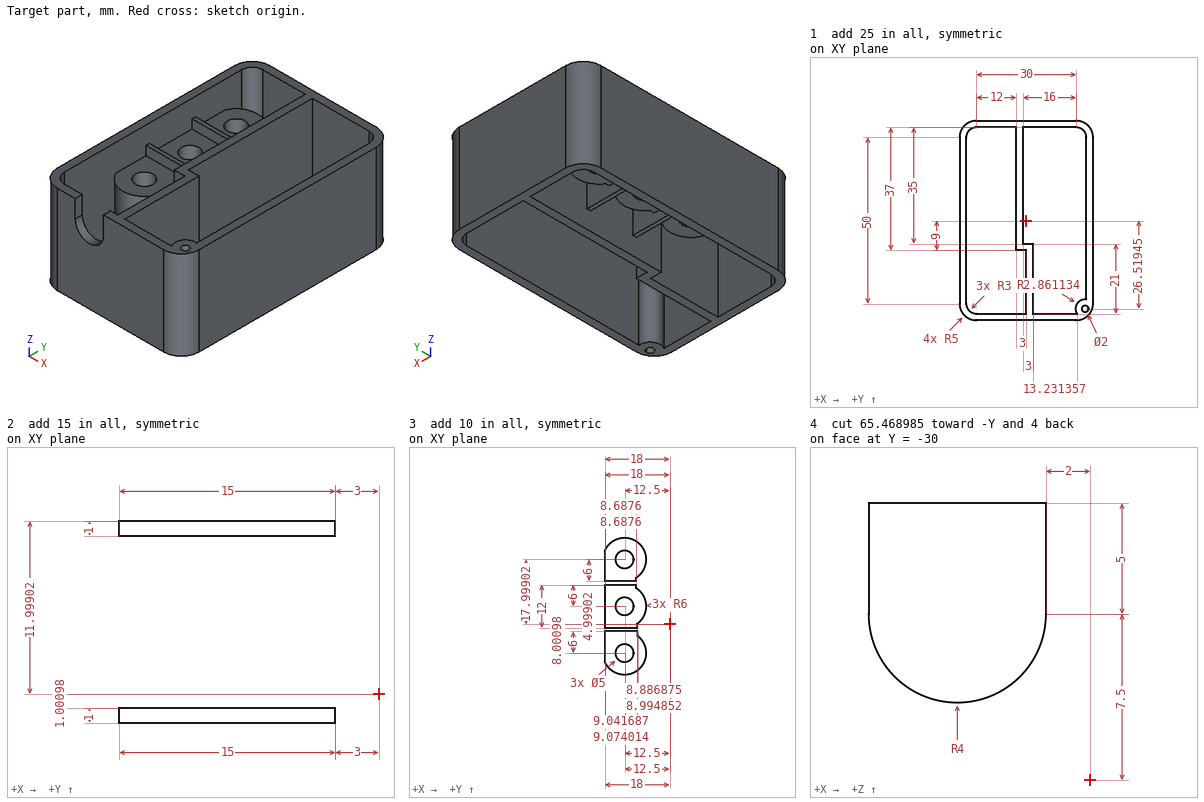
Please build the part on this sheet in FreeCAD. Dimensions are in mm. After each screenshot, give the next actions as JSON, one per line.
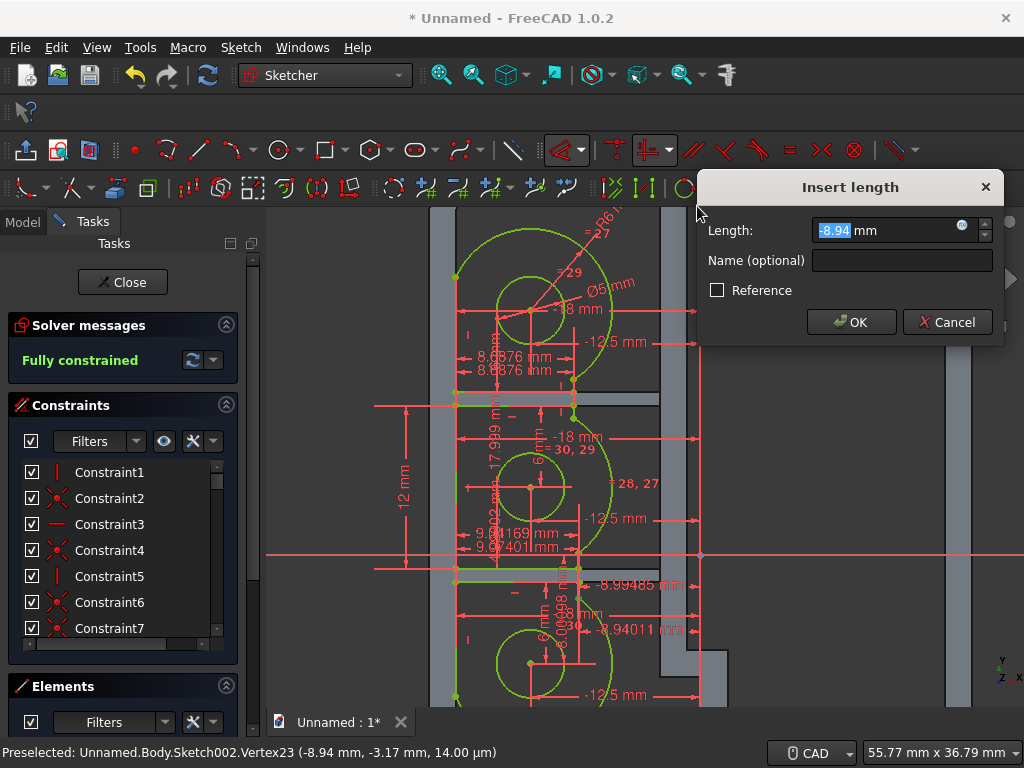
{"action": "type", "text": "-8.886875"}
{"action": "key", "text": "Return"}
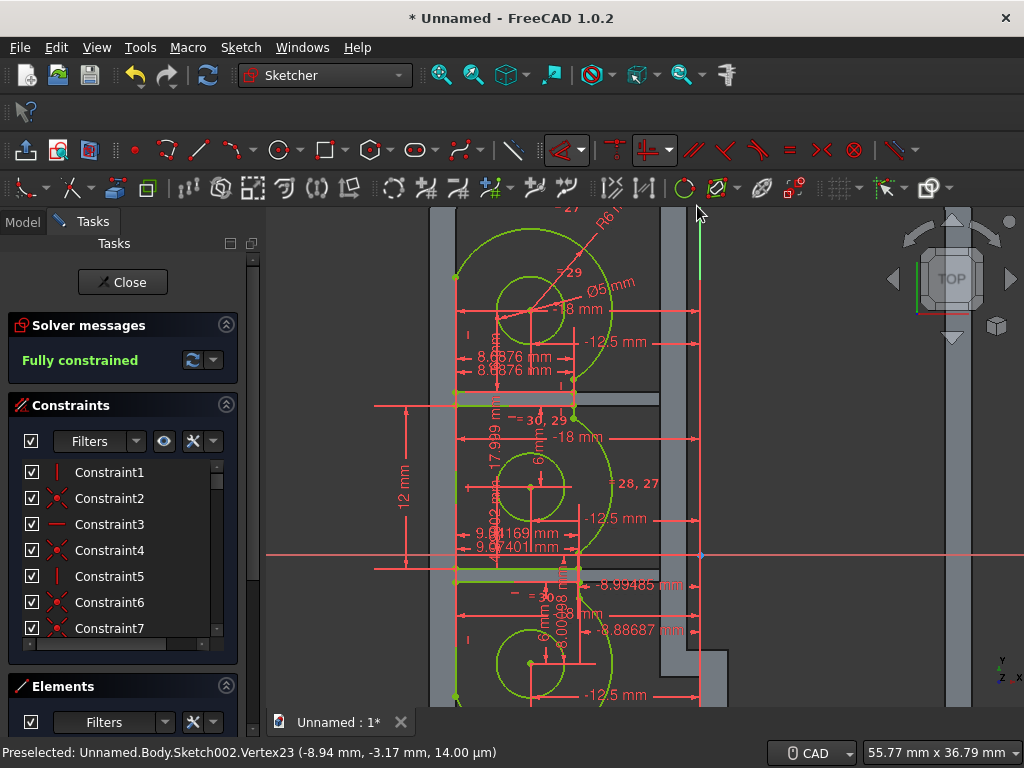
{"action": "left_click", "coordinate": [123, 282]}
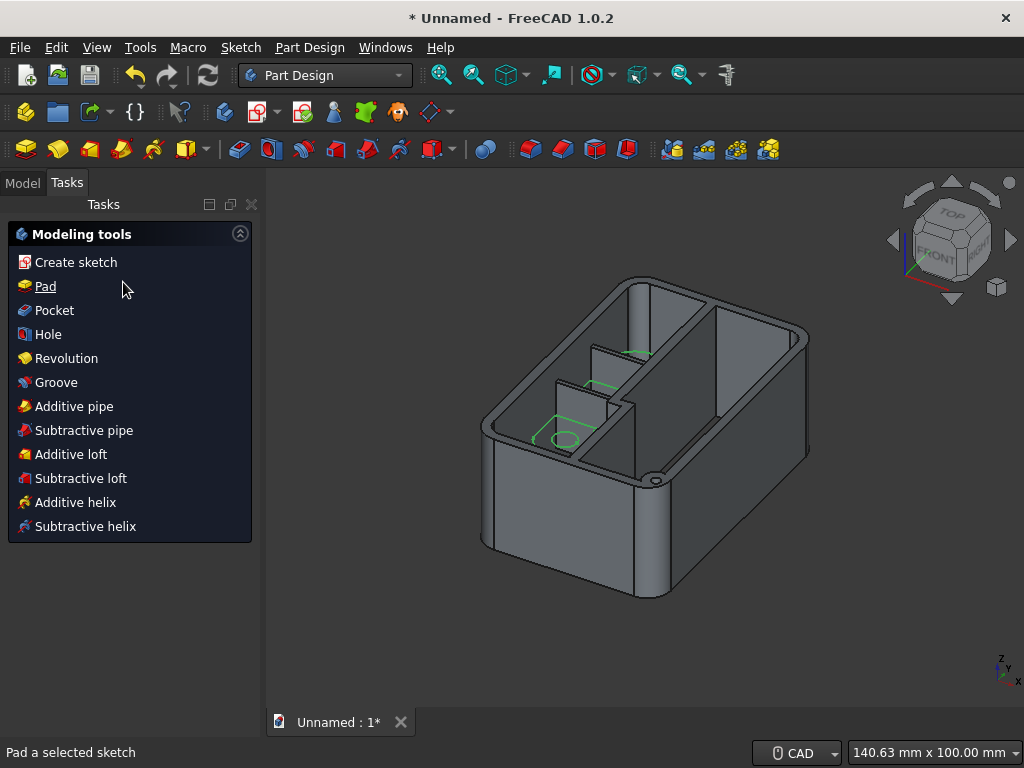
{"action": "left_click", "coordinate": [26, 150]}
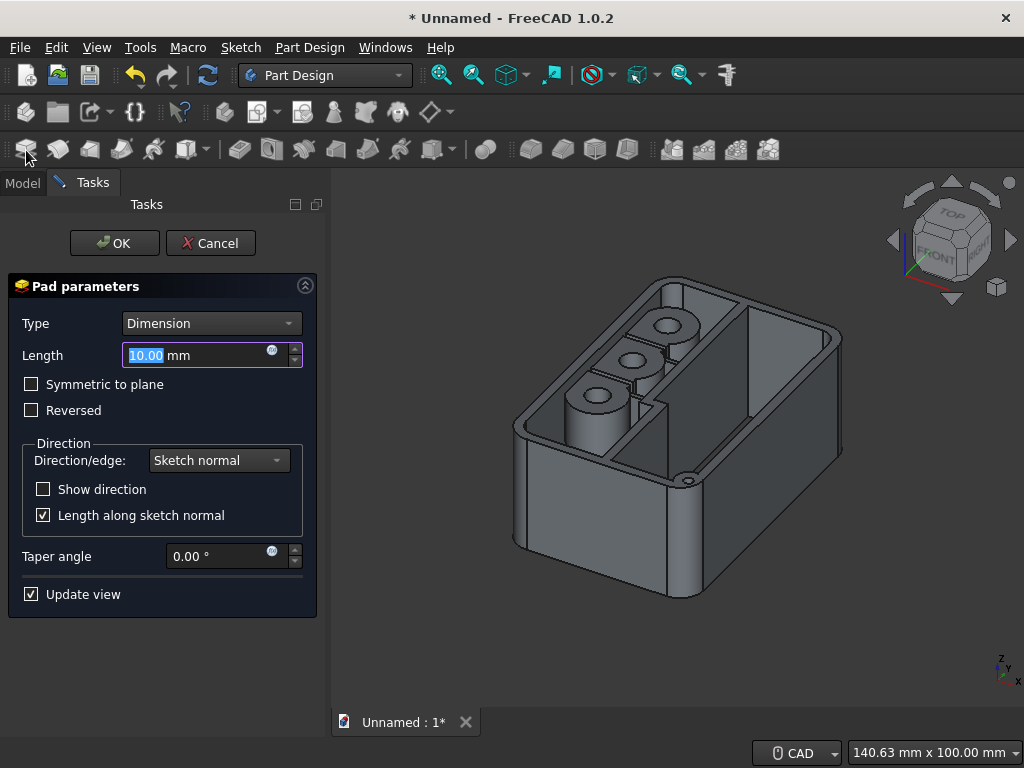
{"action": "type", "text": "10"}
{"action": "key", "text": "Tab"}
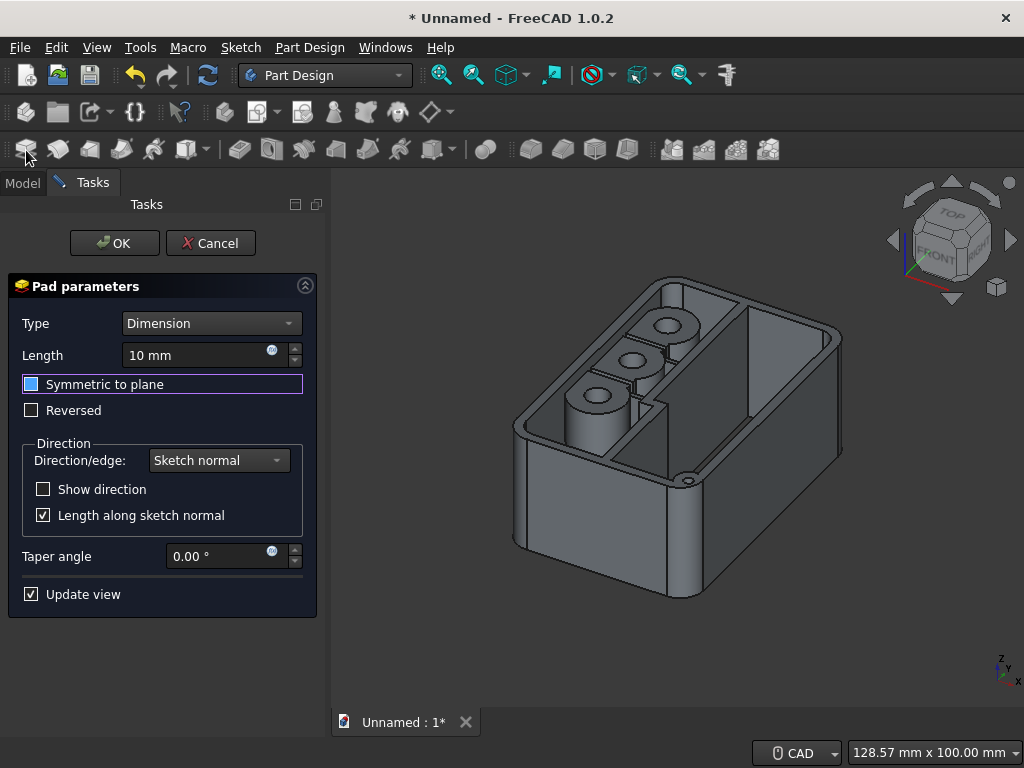
{"action": "left_click", "coordinate": [30, 384]}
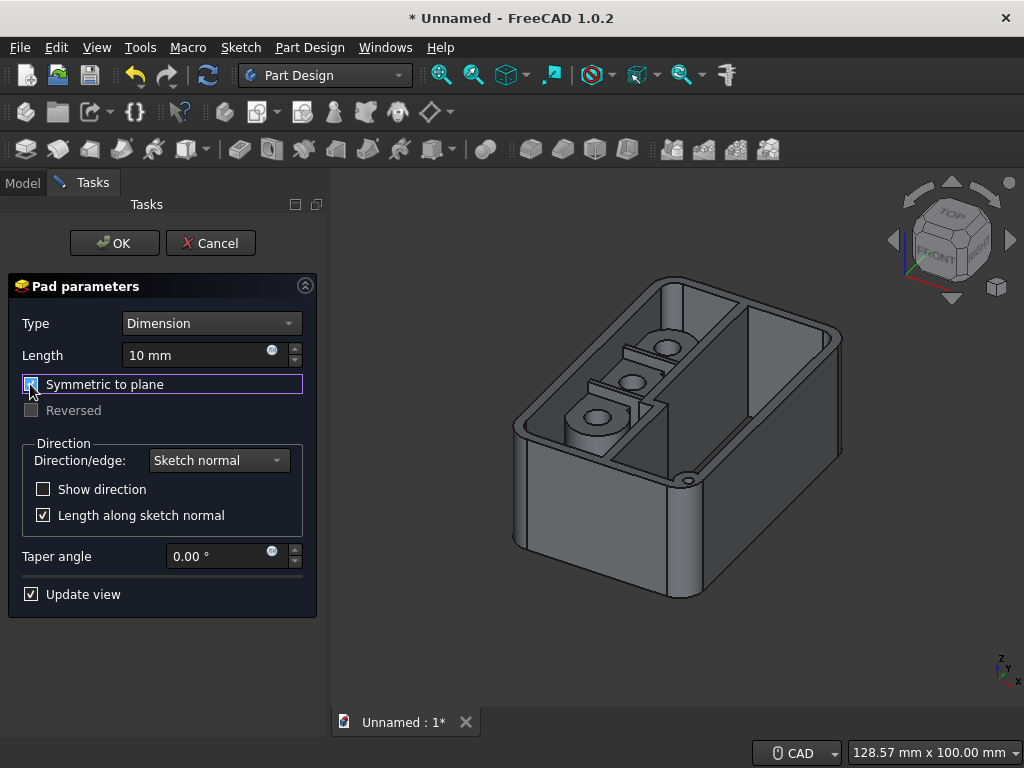
{"action": "left_click", "coordinate": [115, 243]}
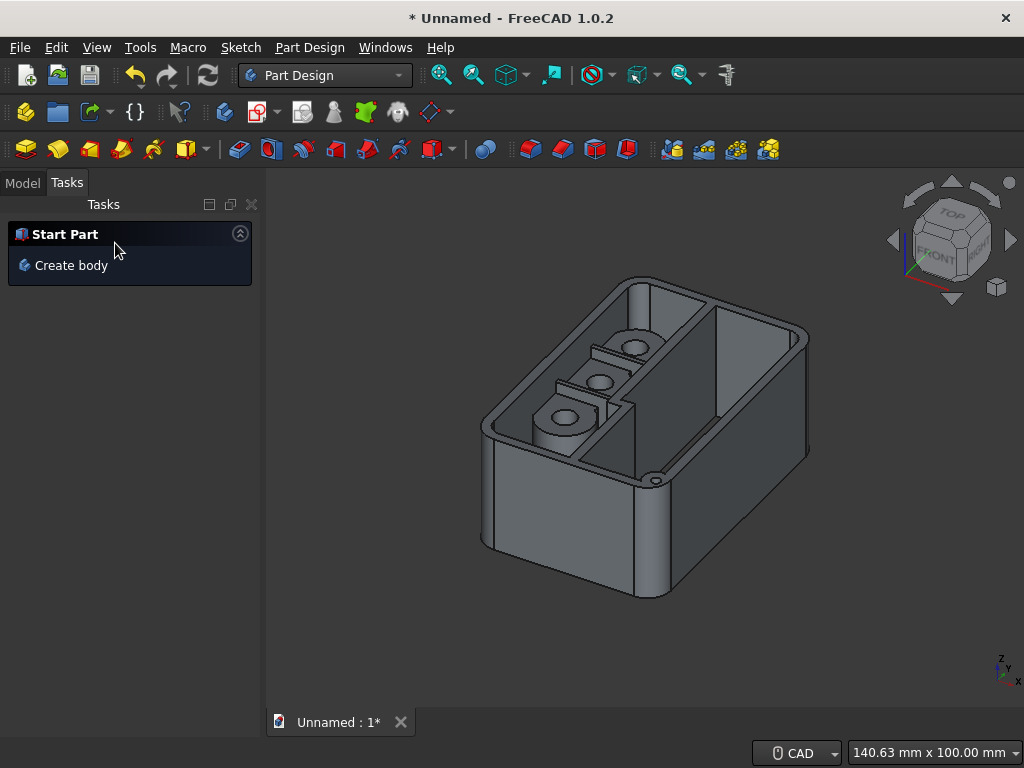
{"action": "left_click", "coordinate": [564, 517]}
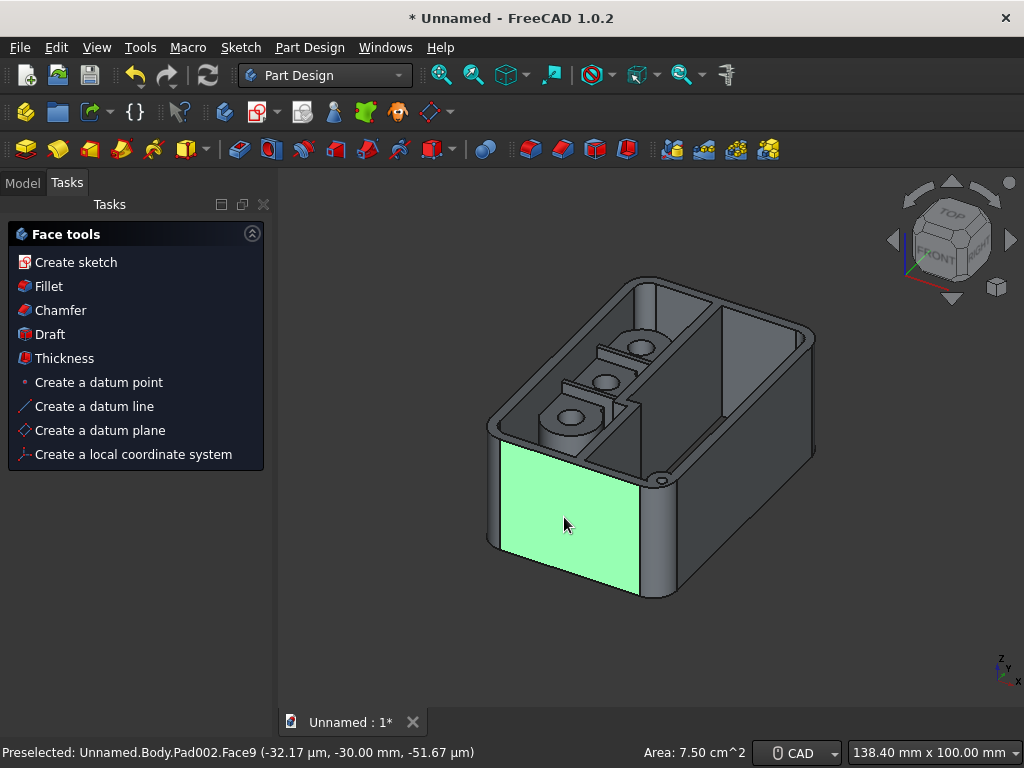
{"action": "left_click", "coordinate": [258, 112]}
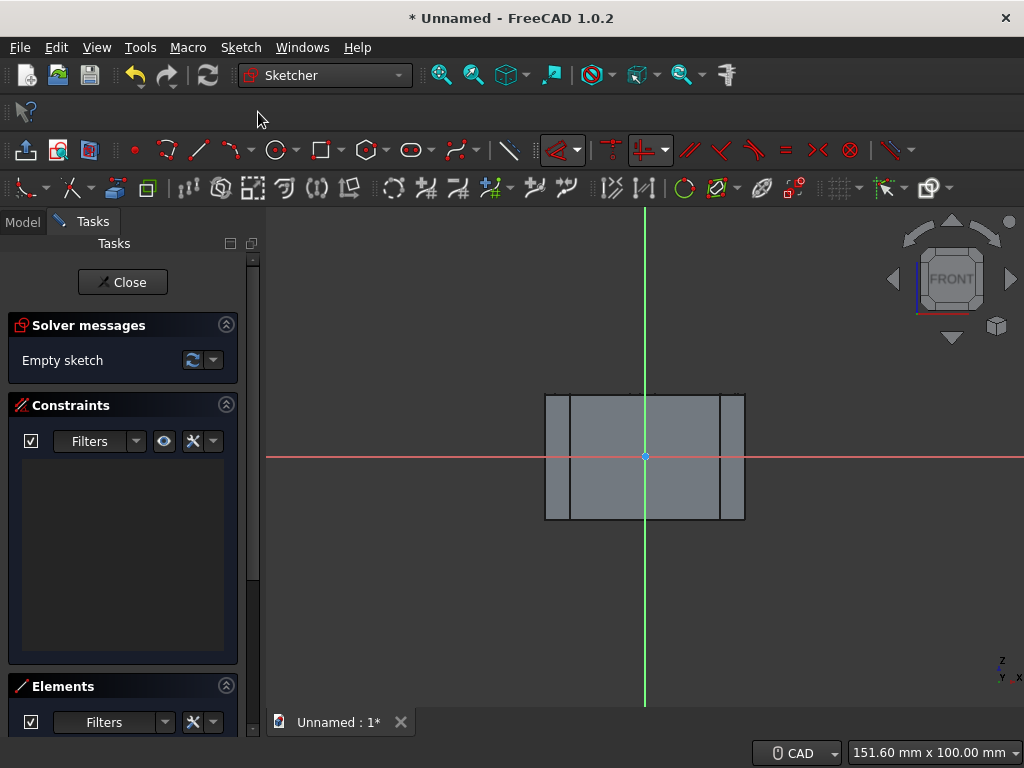
{"action": "scroll", "coordinate": [631, 418], "scroll_direction": "up", "scroll_amount": 8}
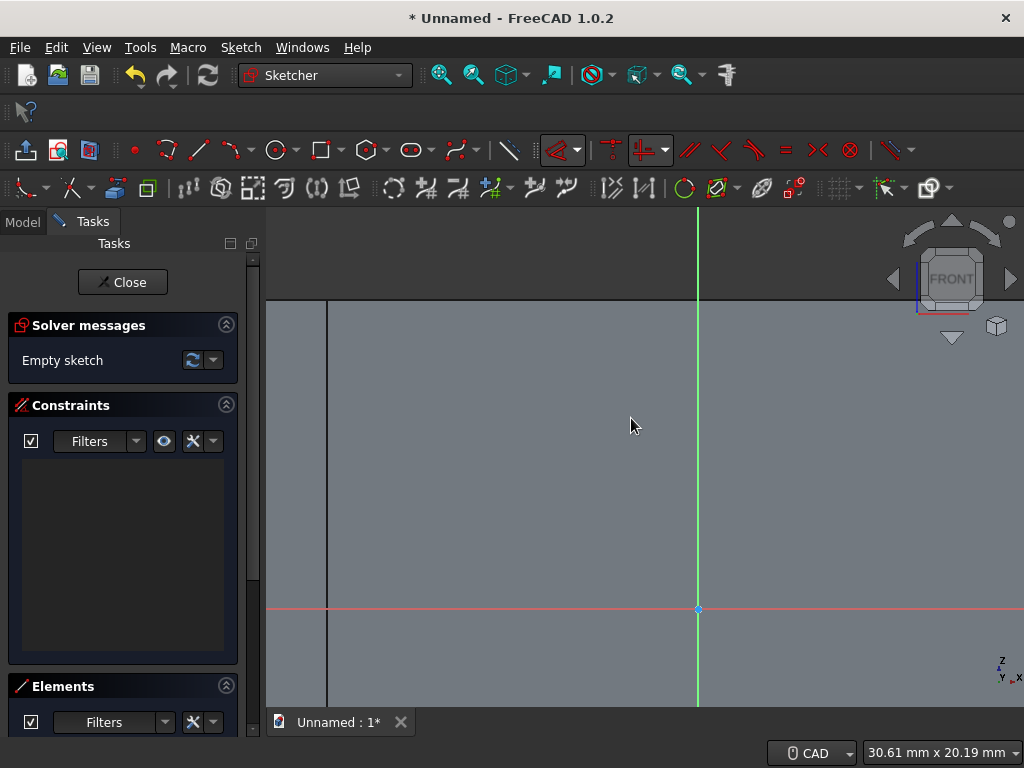
{"action": "left_click", "coordinate": [168, 150]}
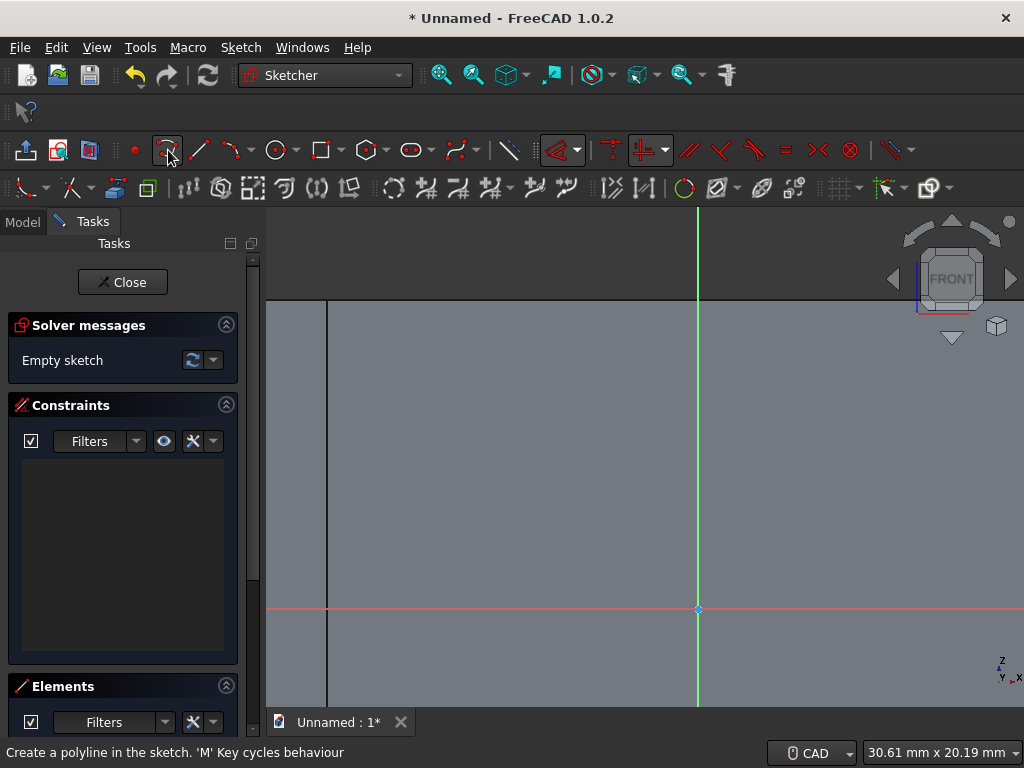
{"action": "left_click", "coordinate": [649, 424]}
{"action": "left_click", "coordinate": [649, 300]}
{"action": "left_click", "coordinate": [451, 300]}
{"action": "left_click", "coordinate": [451, 424]}
{"action": "right_click", "coordinate": [451, 424]}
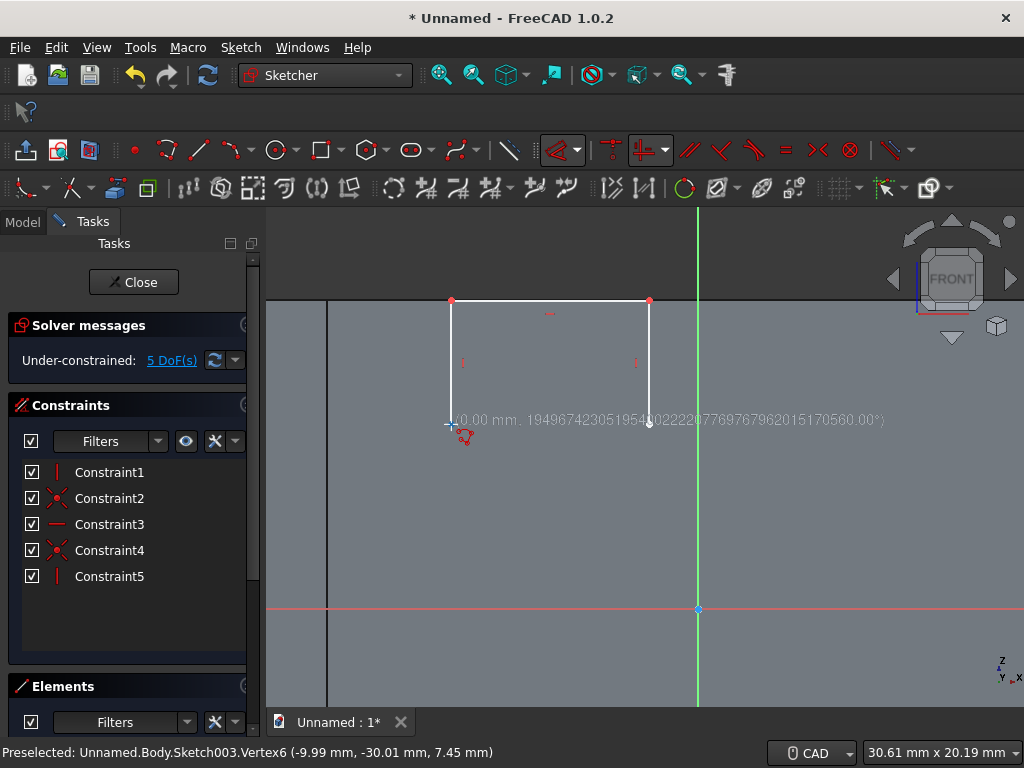
{"action": "left_click", "coordinate": [232, 150]}